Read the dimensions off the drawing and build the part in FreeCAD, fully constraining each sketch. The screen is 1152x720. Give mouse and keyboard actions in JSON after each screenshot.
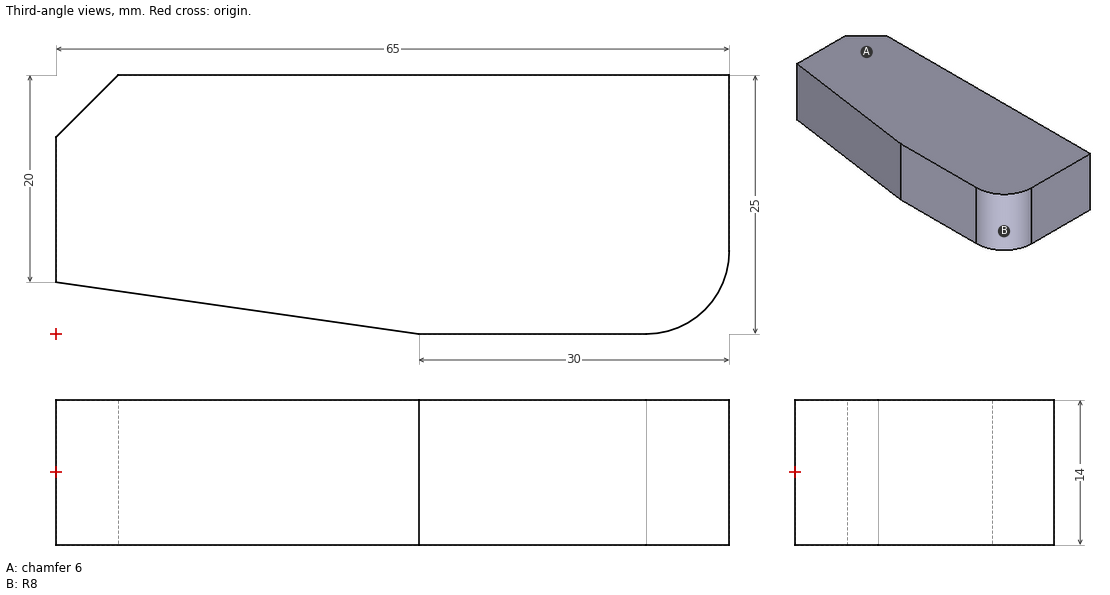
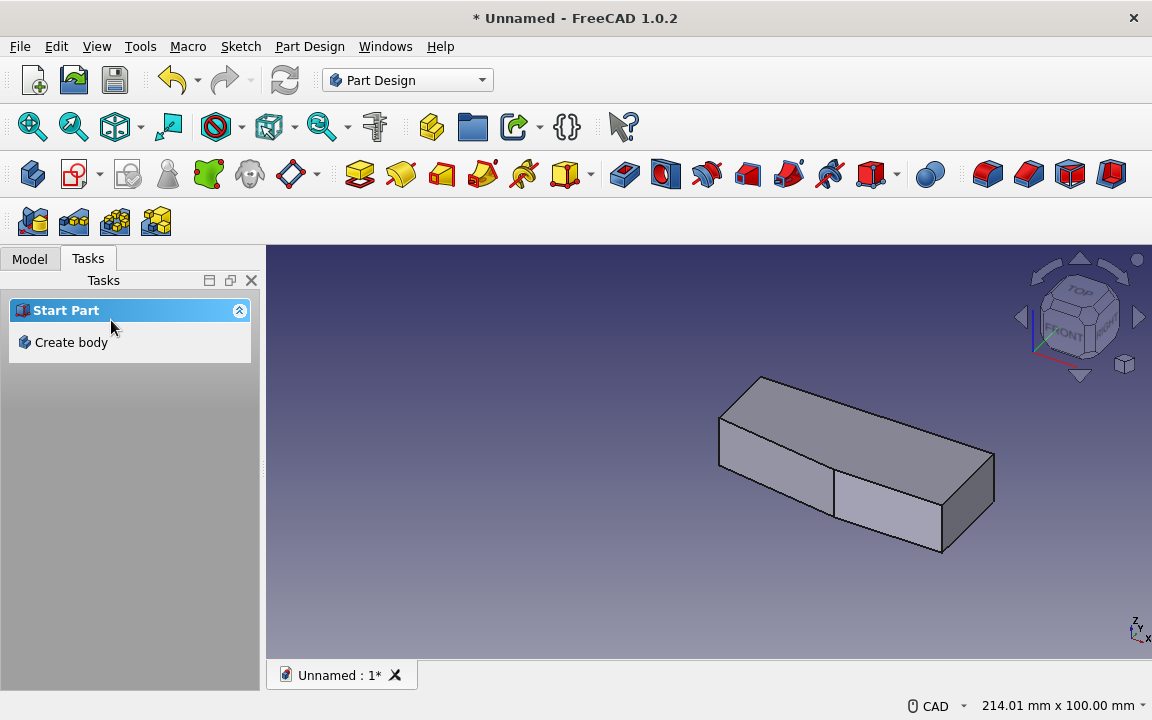
{"action": "left_click", "coordinate": [33, 128]}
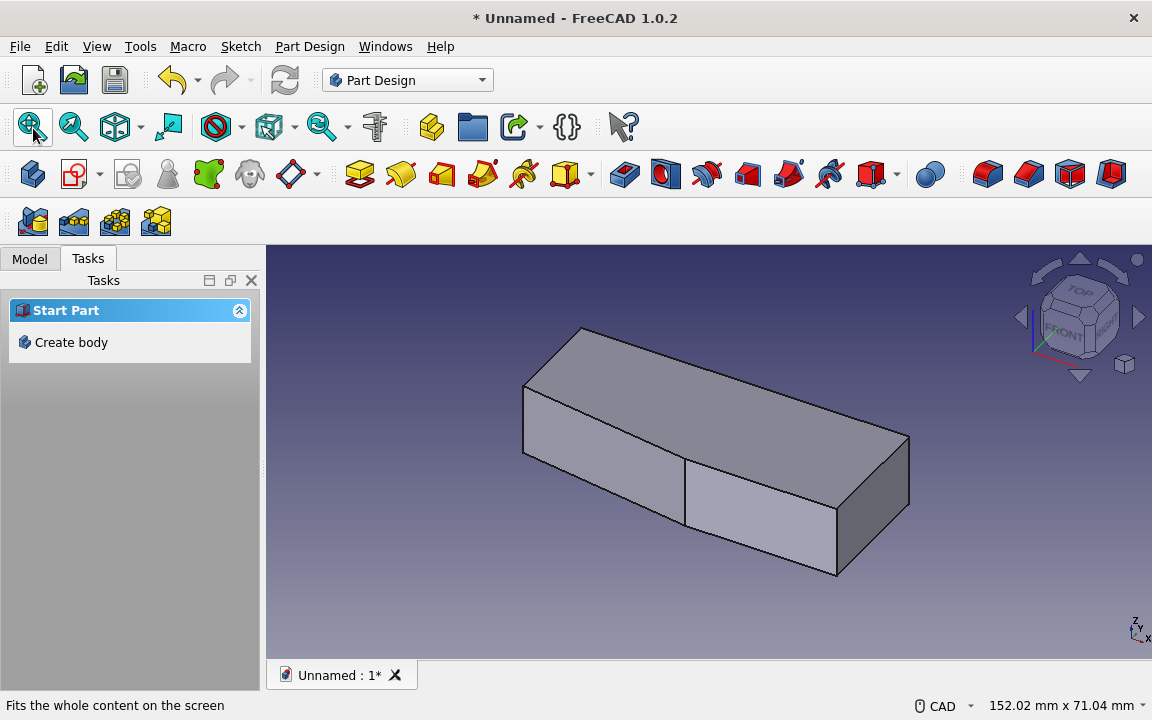
{"action": "key", "text": "0"}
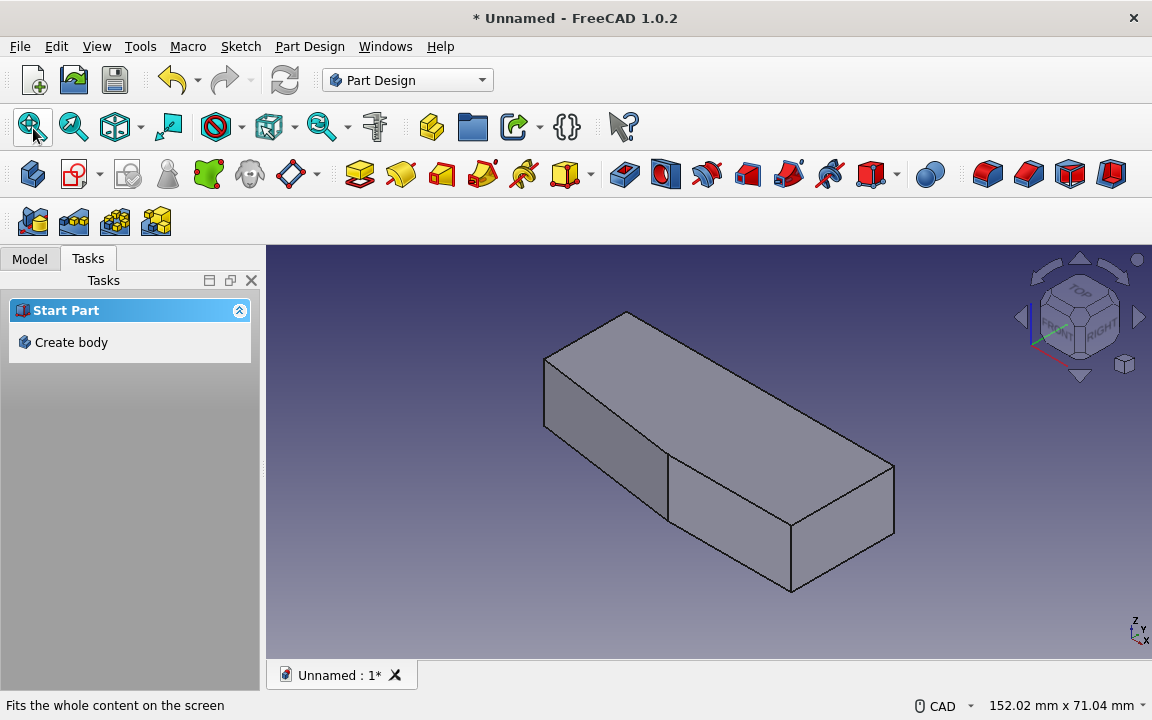
{"action": "key", "text": "2"}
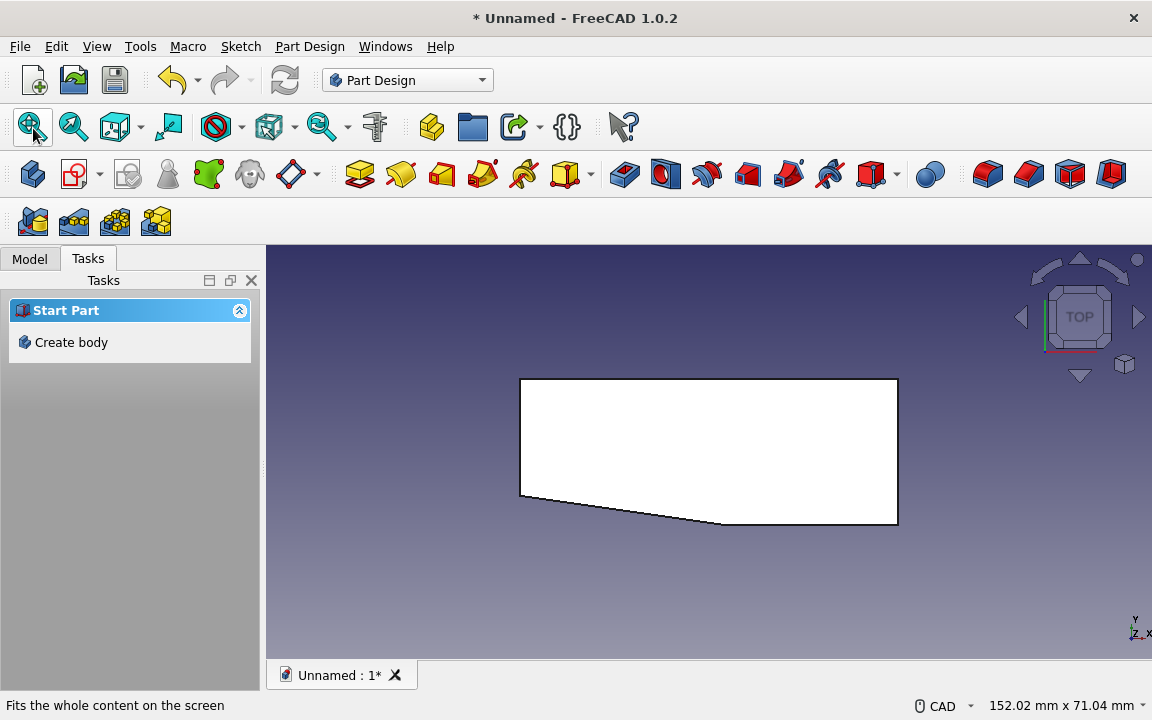
{"action": "left_click", "coordinate": [33, 128]}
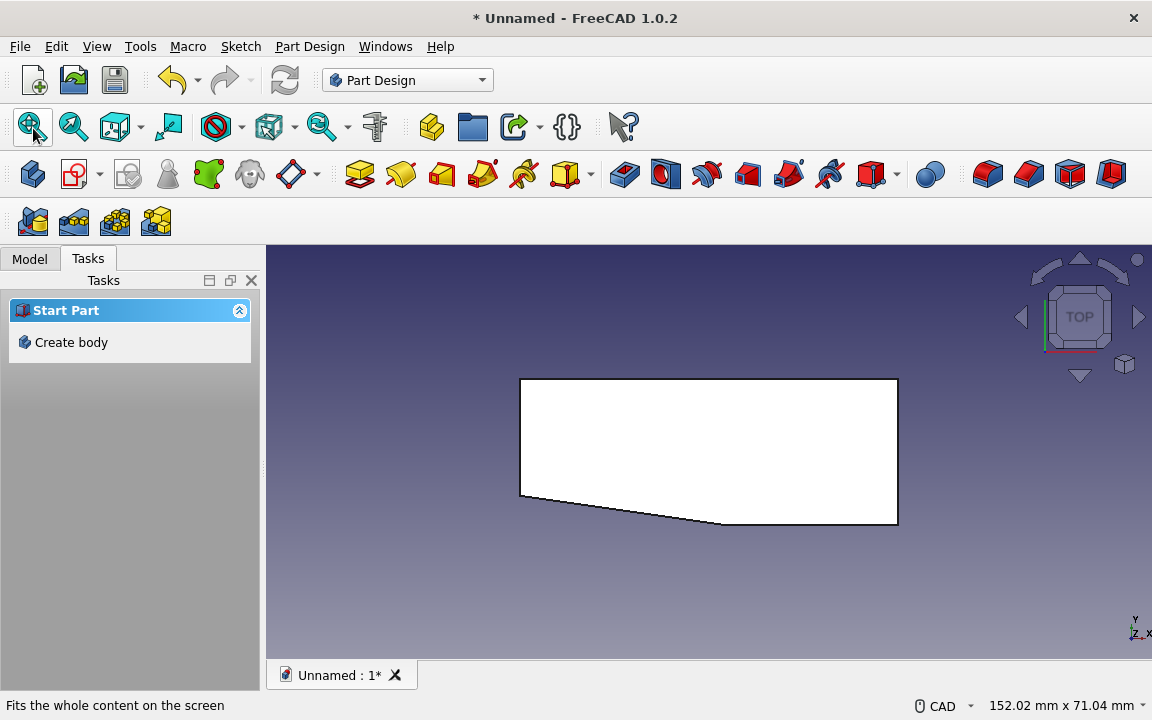
{"action": "key", "text": "1"}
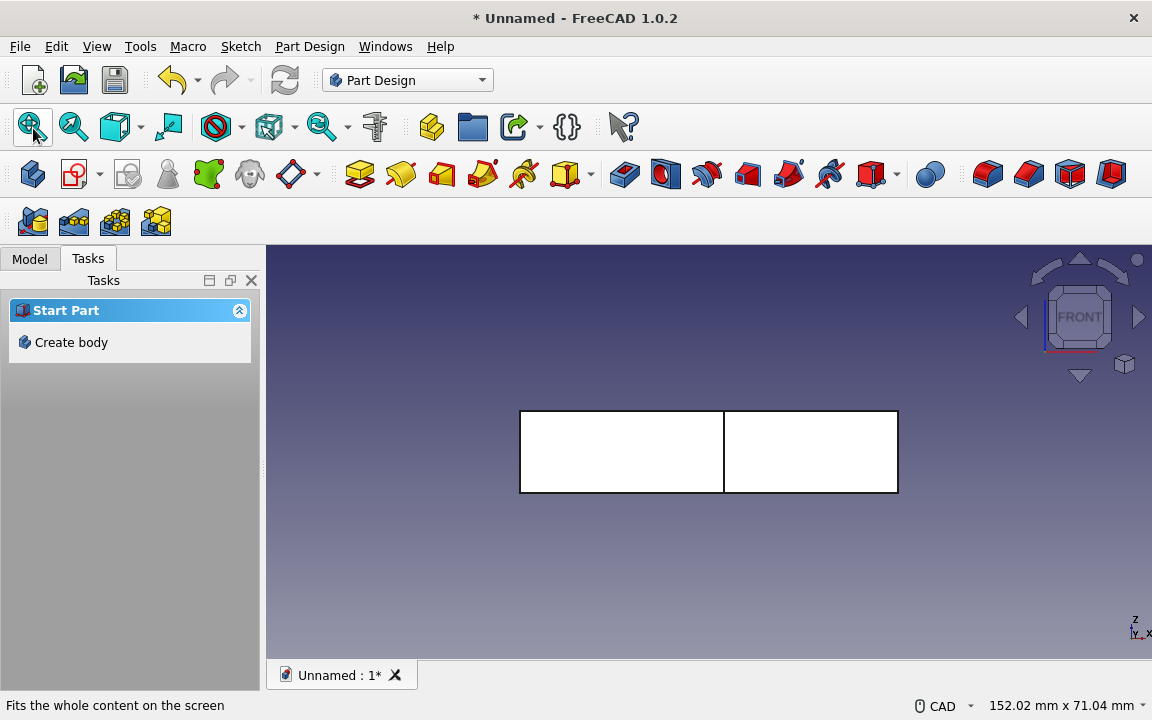
{"action": "left_click", "coordinate": [33, 128]}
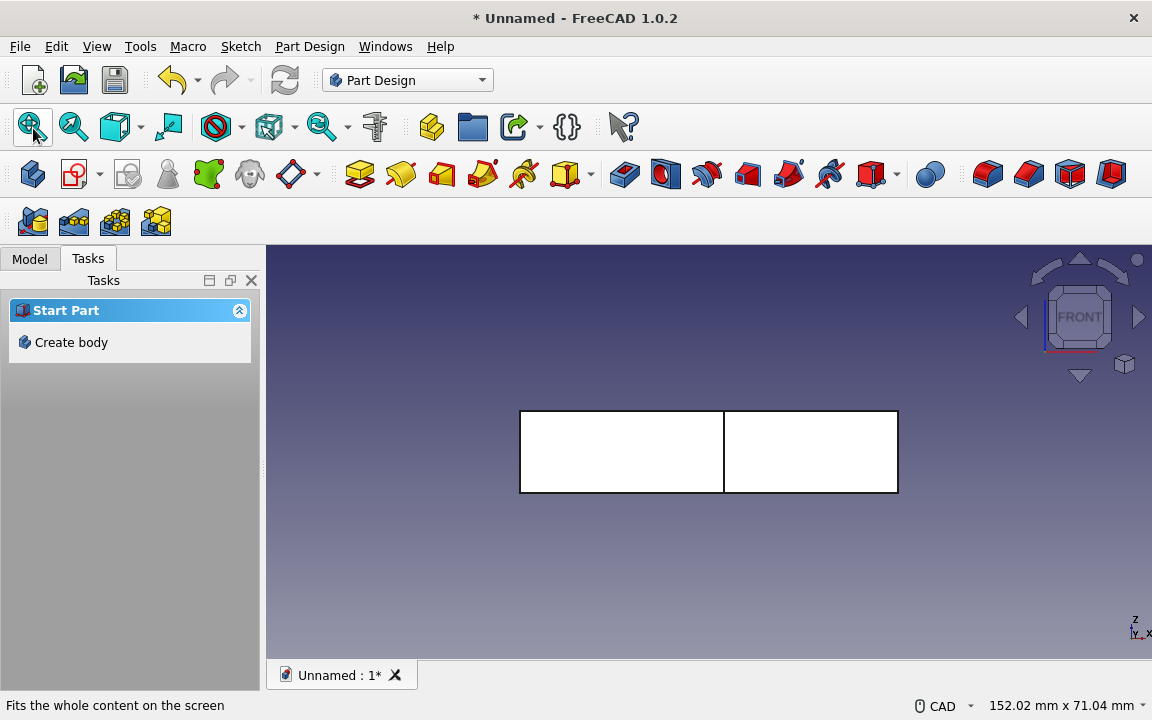
{"action": "key", "text": "3"}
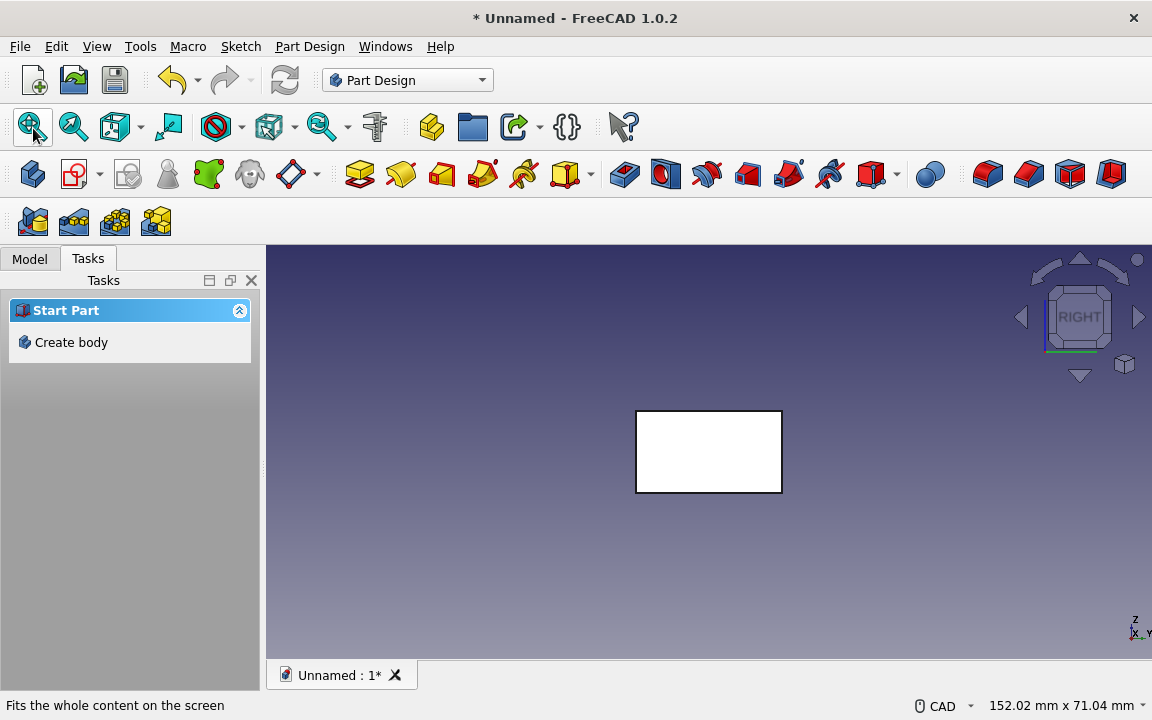
{"action": "left_click", "coordinate": [33, 128]}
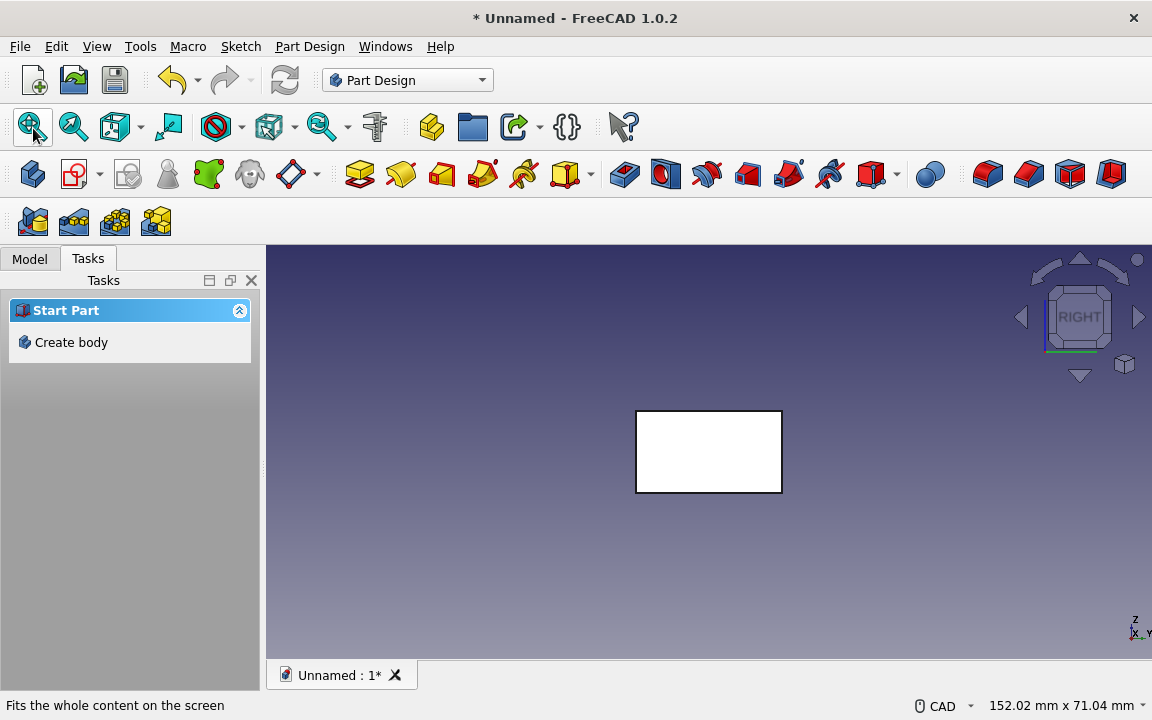
{"action": "key", "text": "5"}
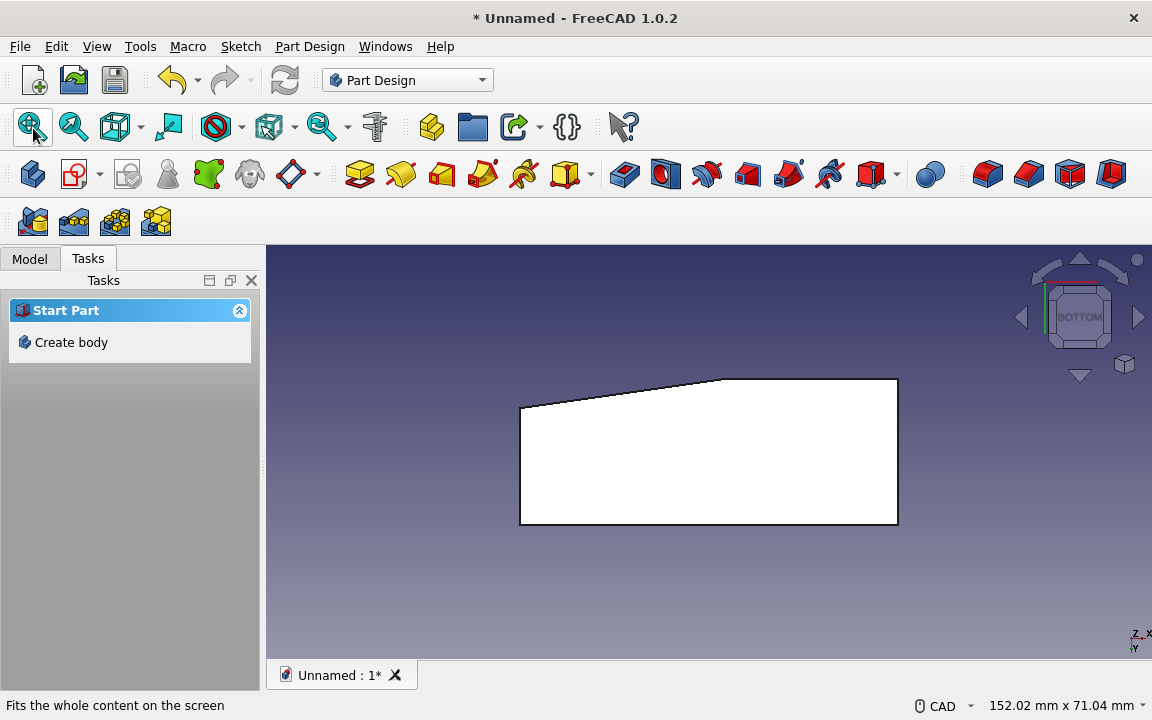
{"action": "left_click", "coordinate": [33, 128]}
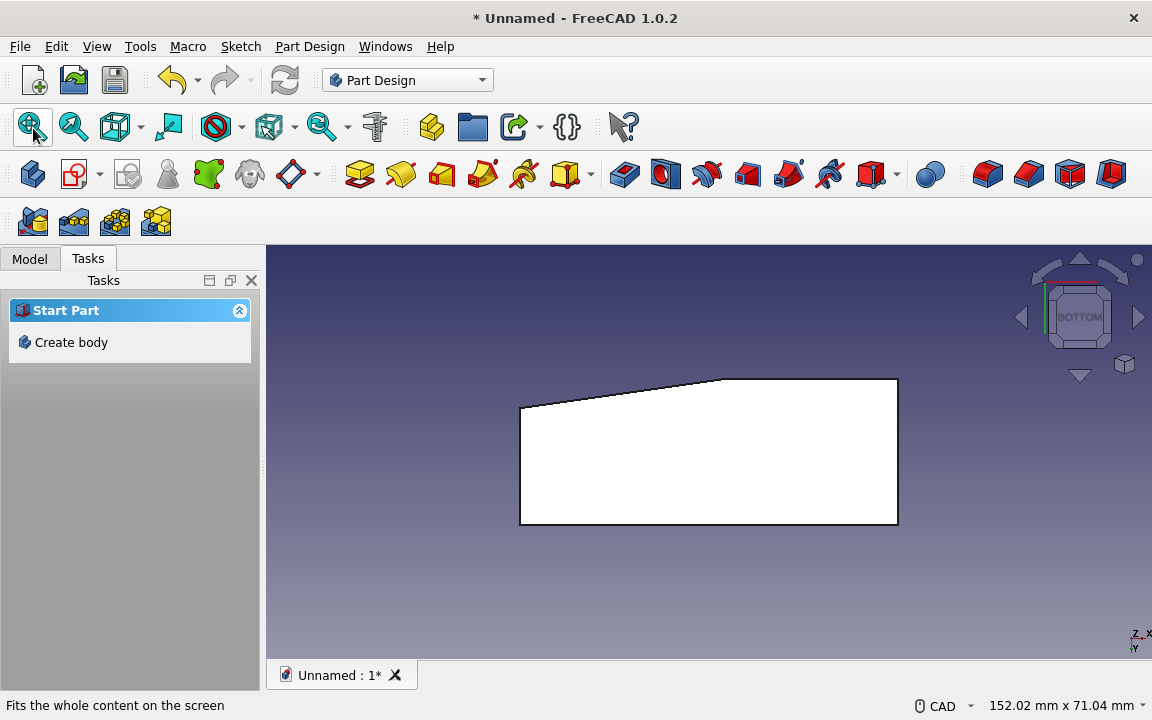
{"action": "key", "text": "4"}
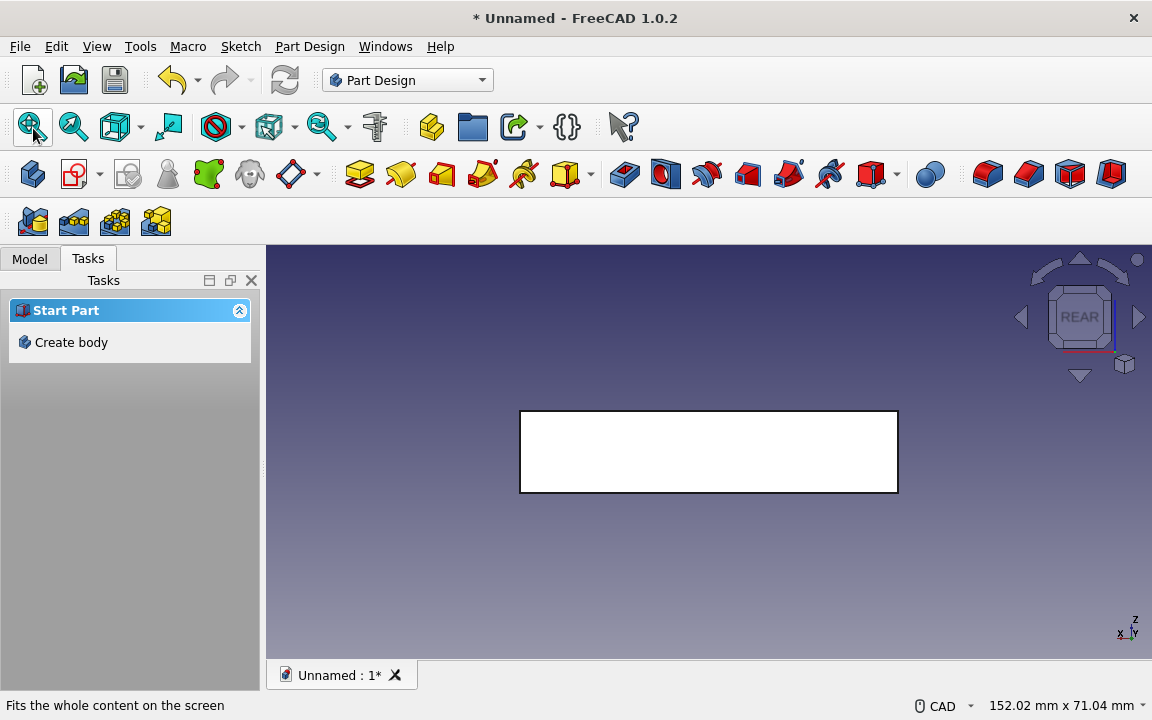
{"action": "left_click", "coordinate": [33, 128]}